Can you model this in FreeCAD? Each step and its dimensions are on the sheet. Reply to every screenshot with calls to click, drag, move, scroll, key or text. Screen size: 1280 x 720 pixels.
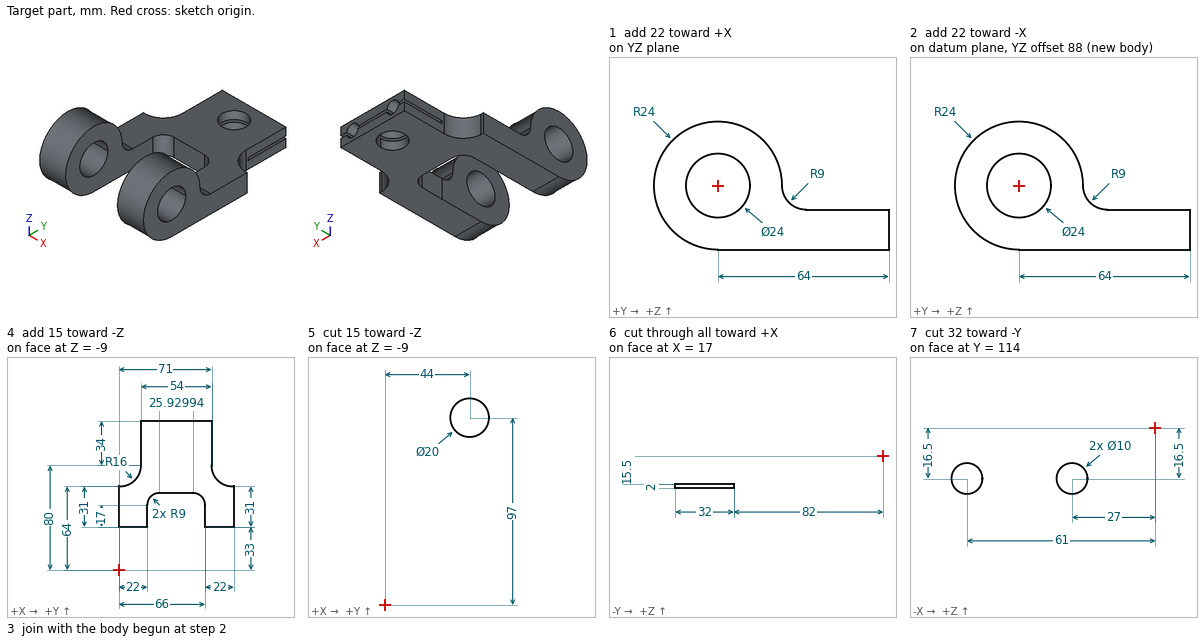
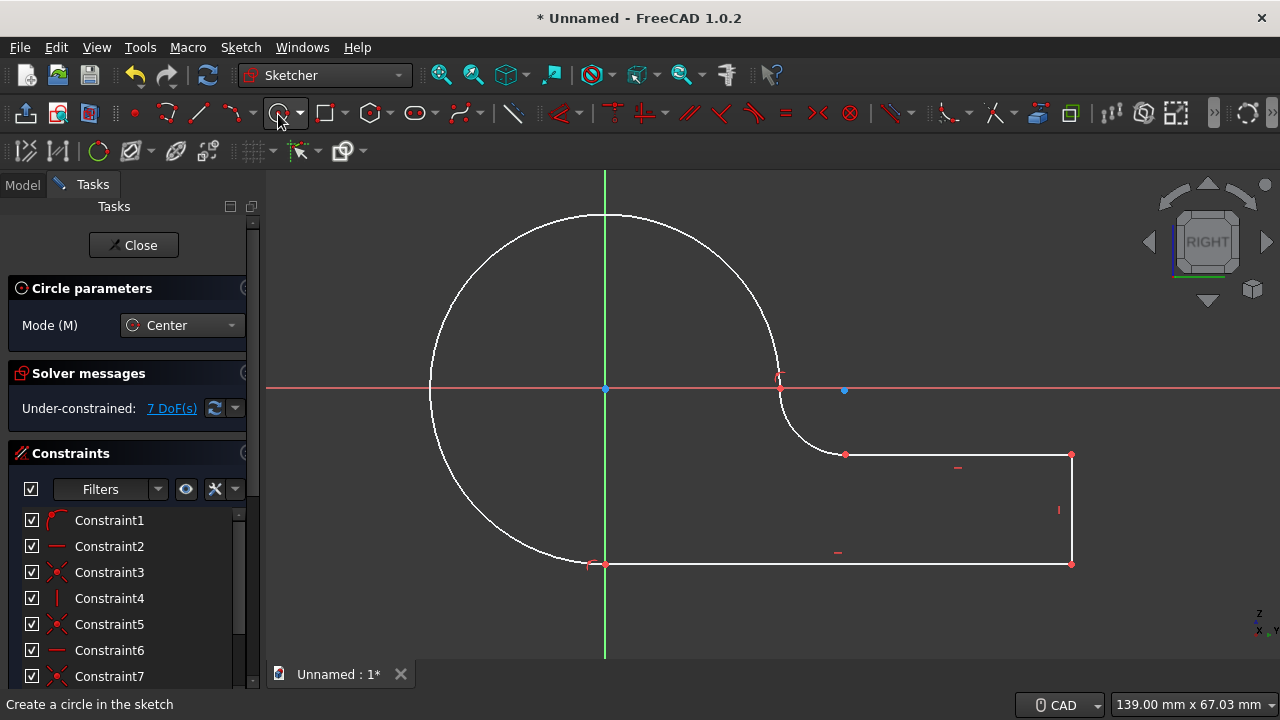
click(605, 388)
click(667, 327)
key(Escape)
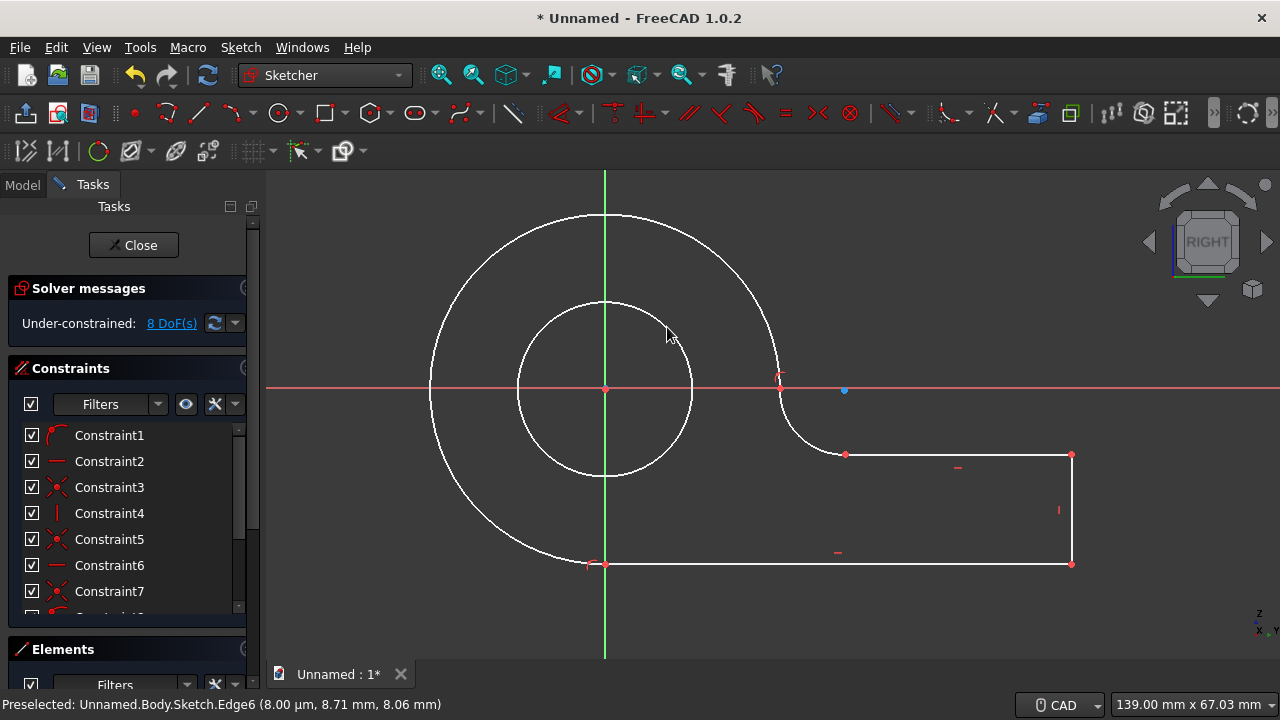
click(745, 564)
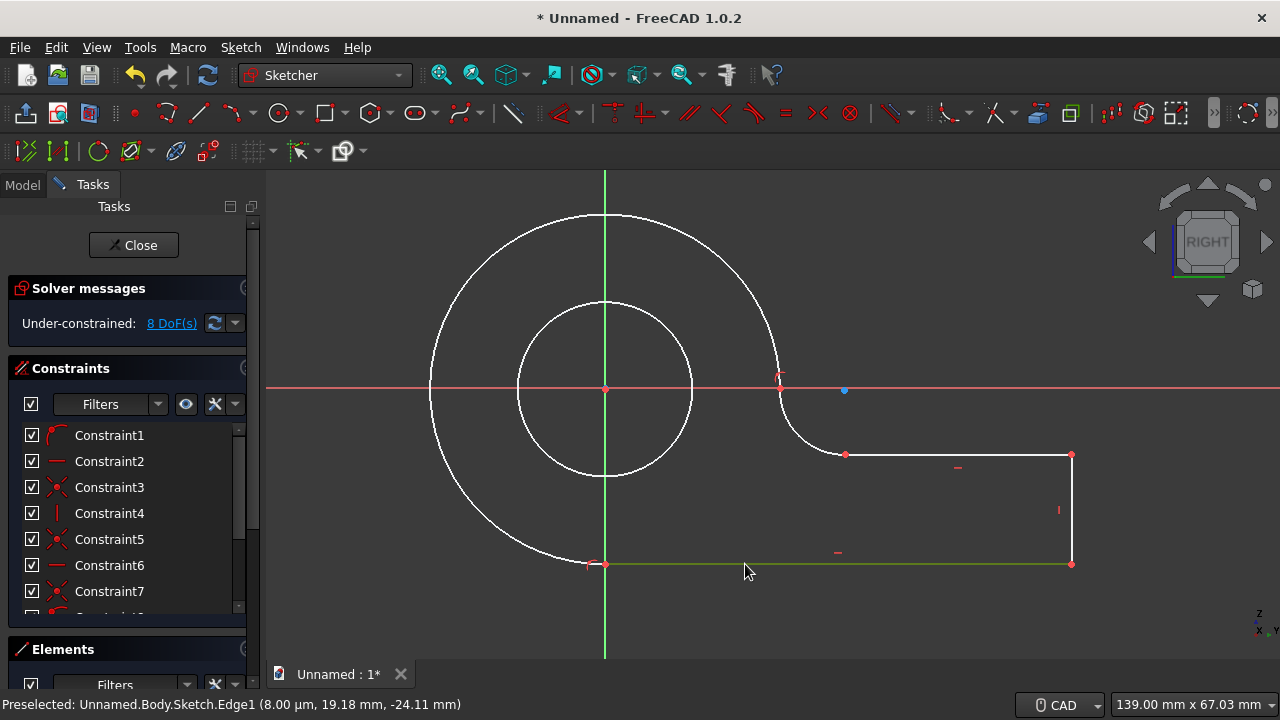
click(632, 216)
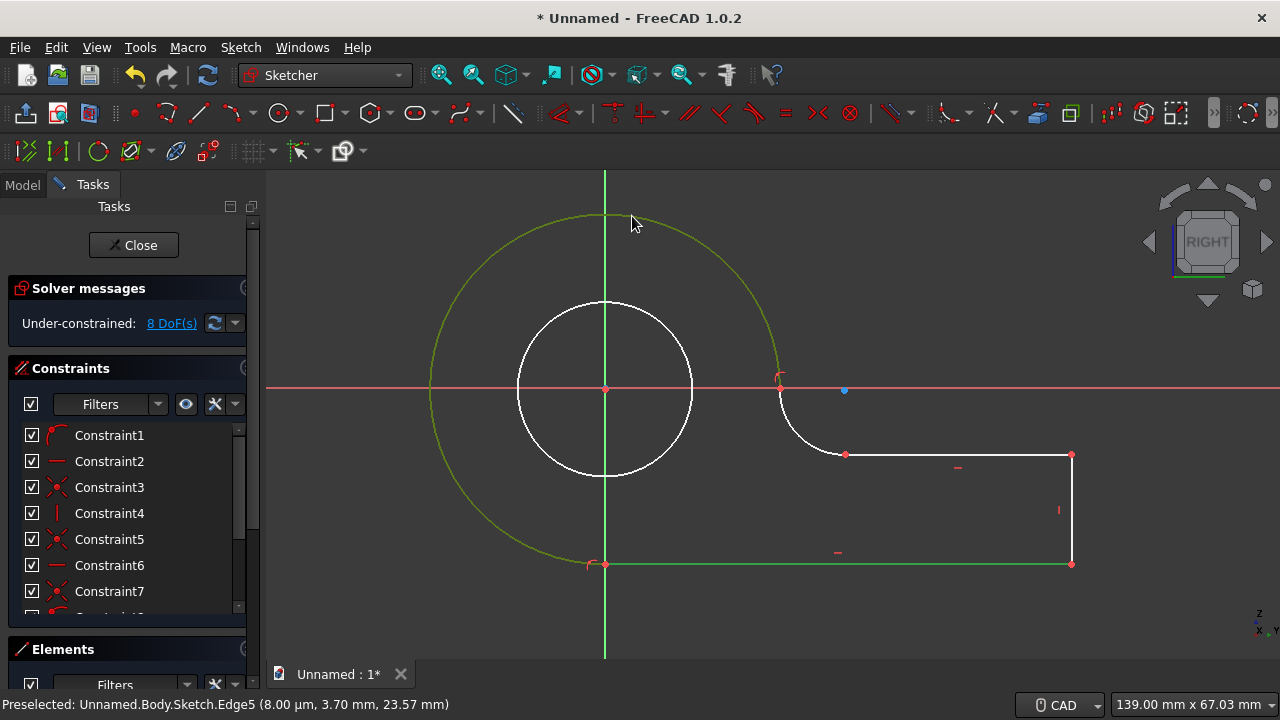
click(754, 114)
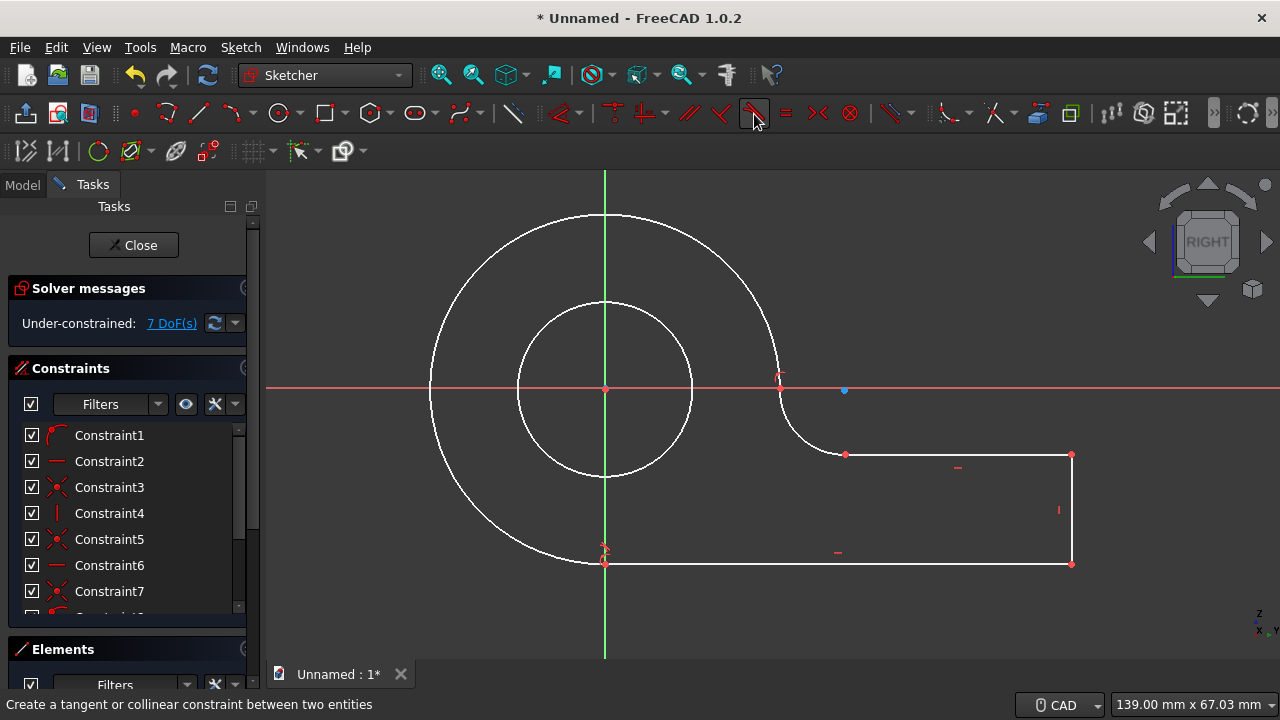
click(1004, 455)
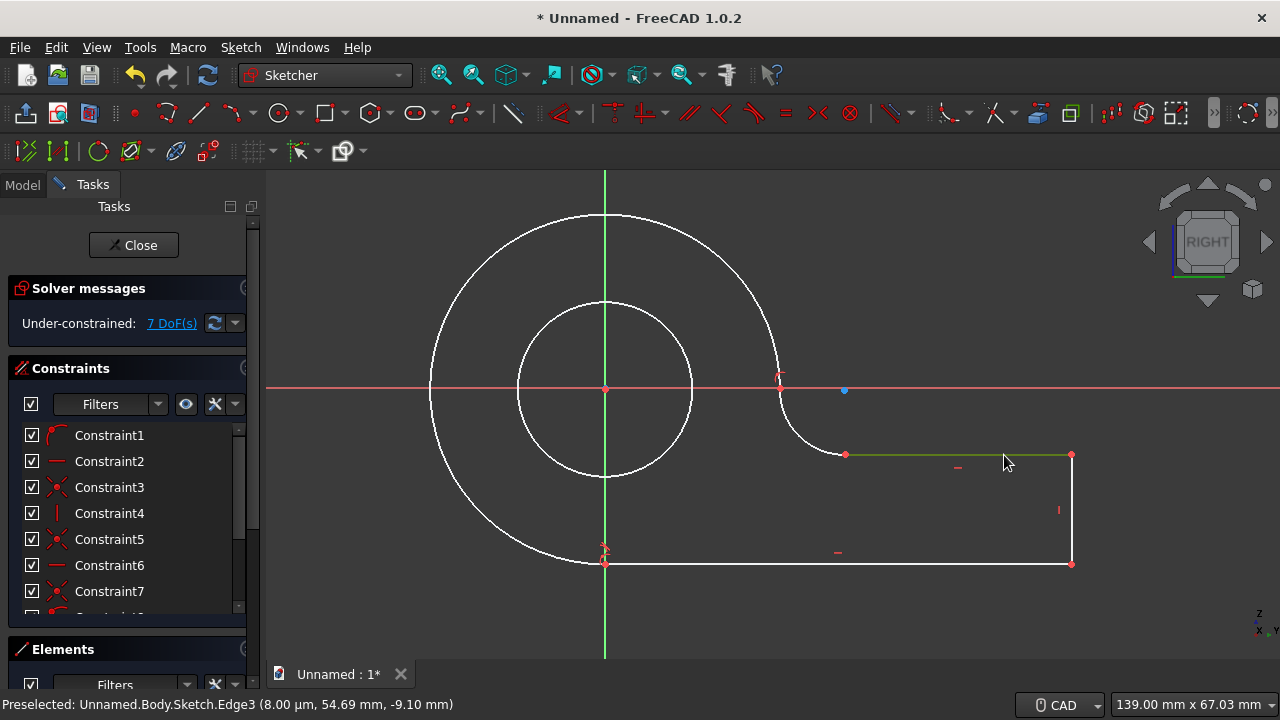
click(787, 419)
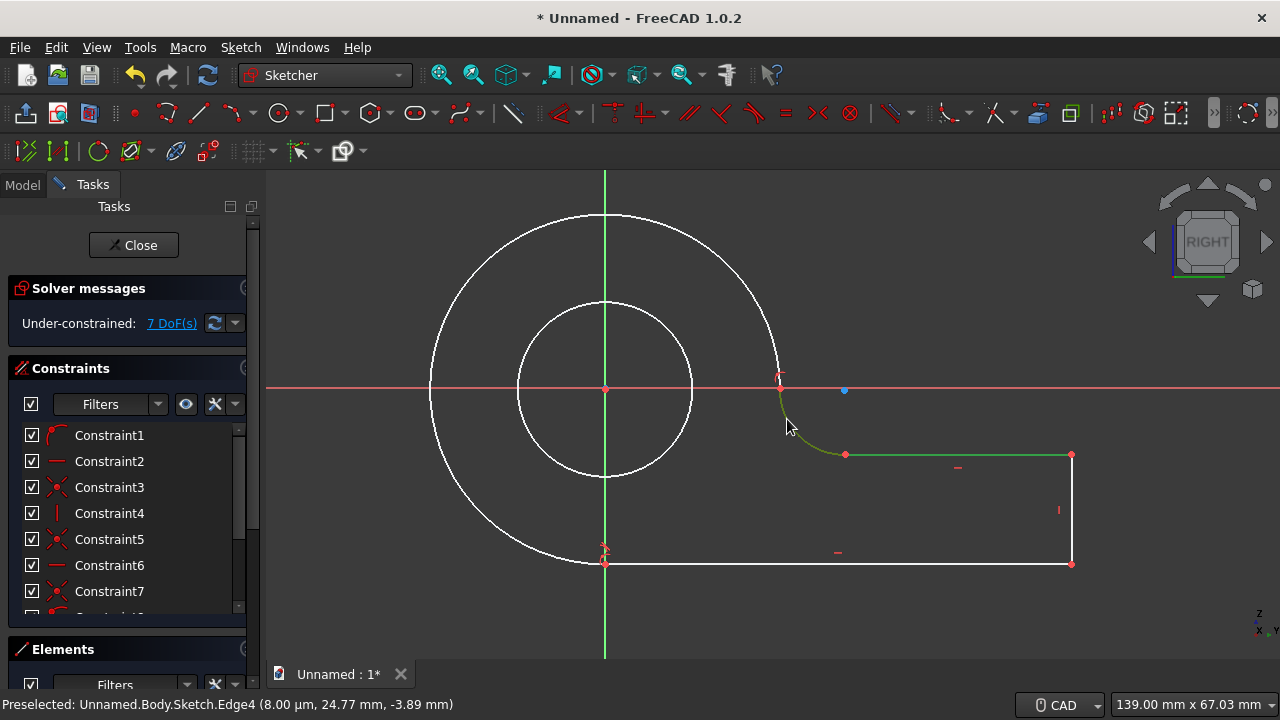
click(754, 114)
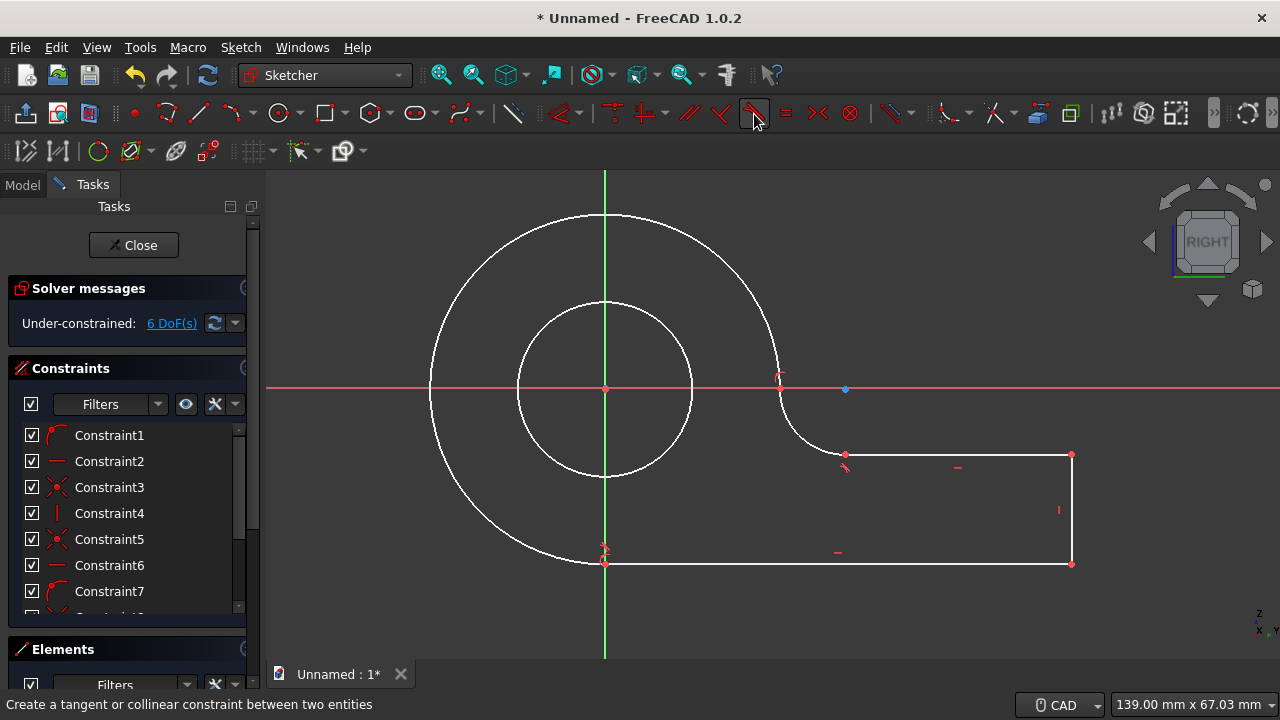
click(787, 419)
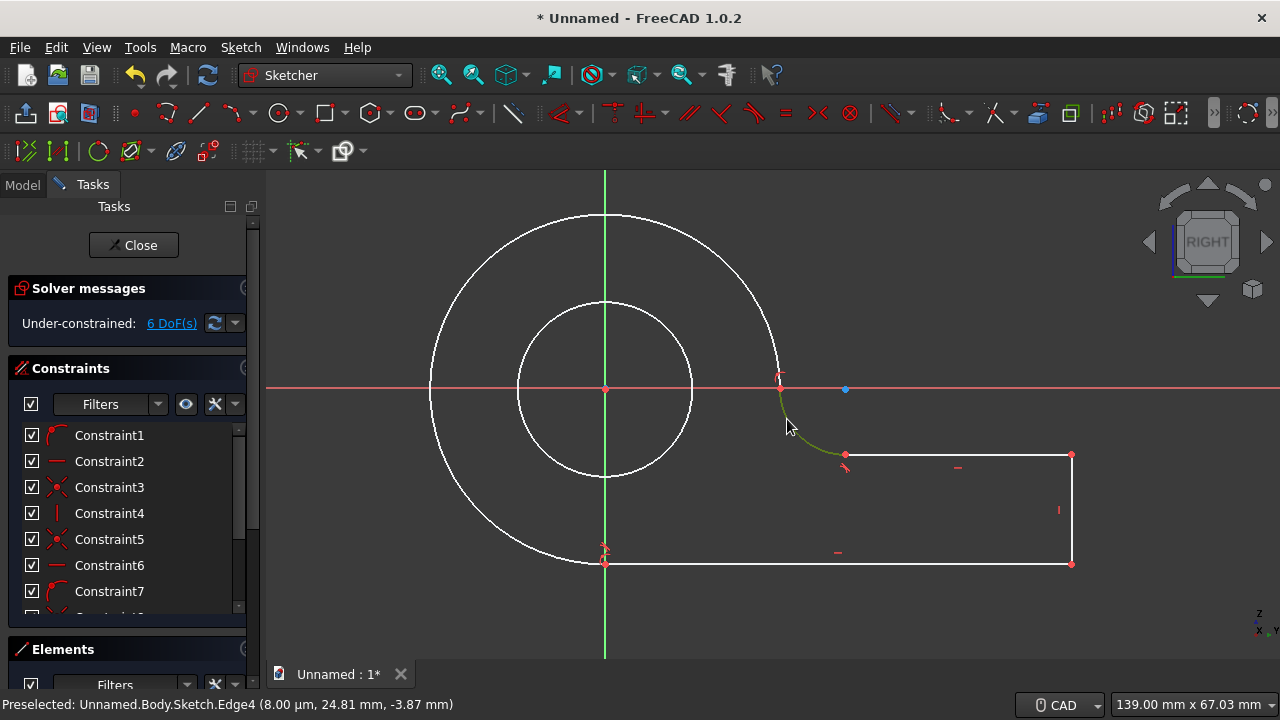
click(632, 217)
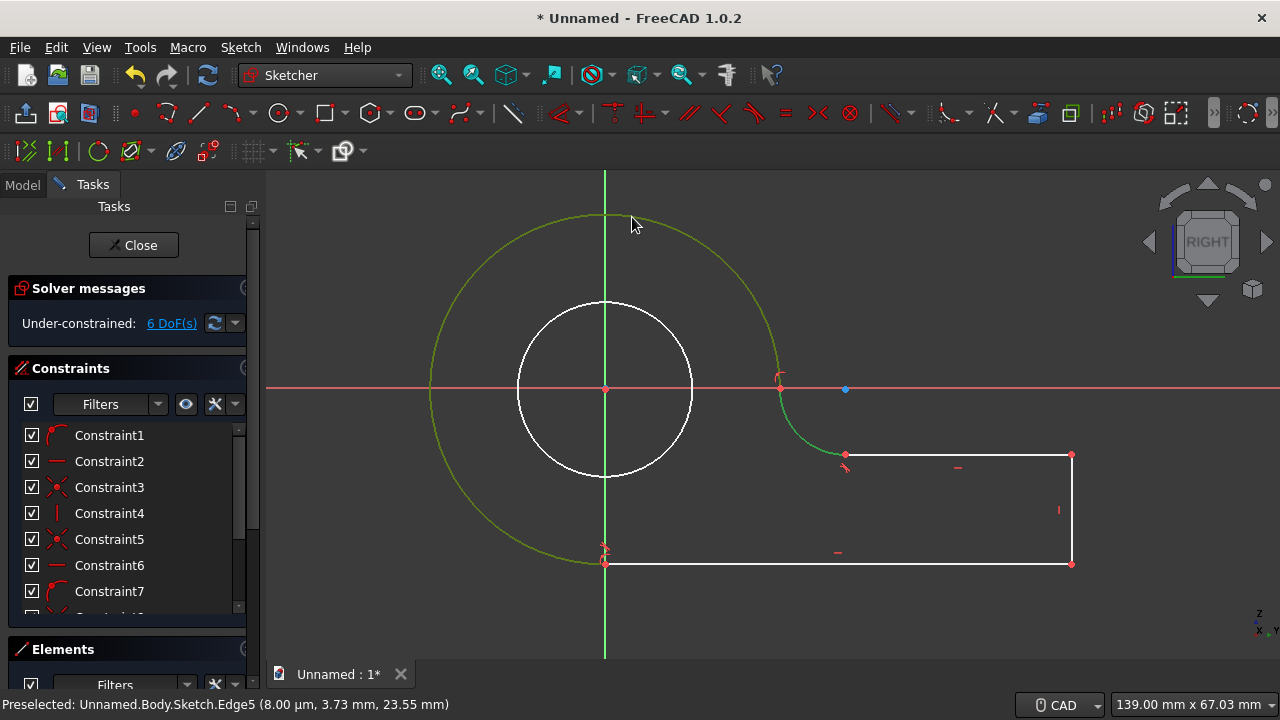
click(754, 114)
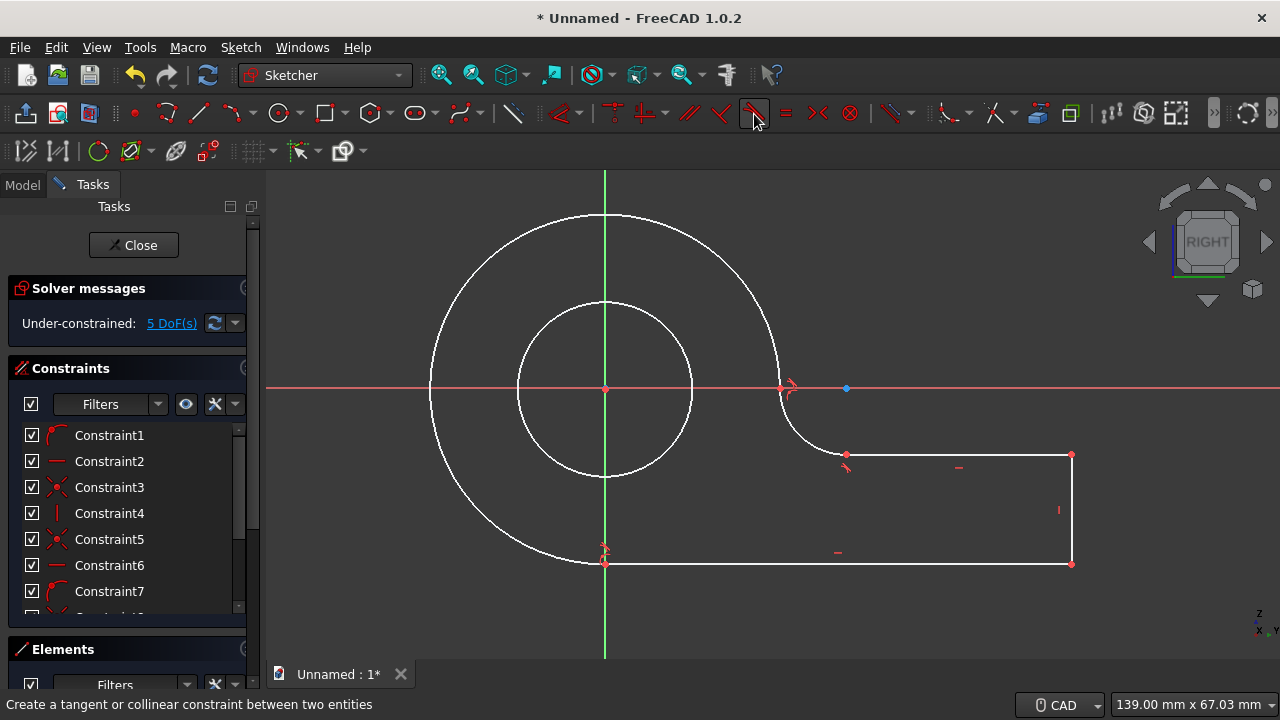
click(847, 388)